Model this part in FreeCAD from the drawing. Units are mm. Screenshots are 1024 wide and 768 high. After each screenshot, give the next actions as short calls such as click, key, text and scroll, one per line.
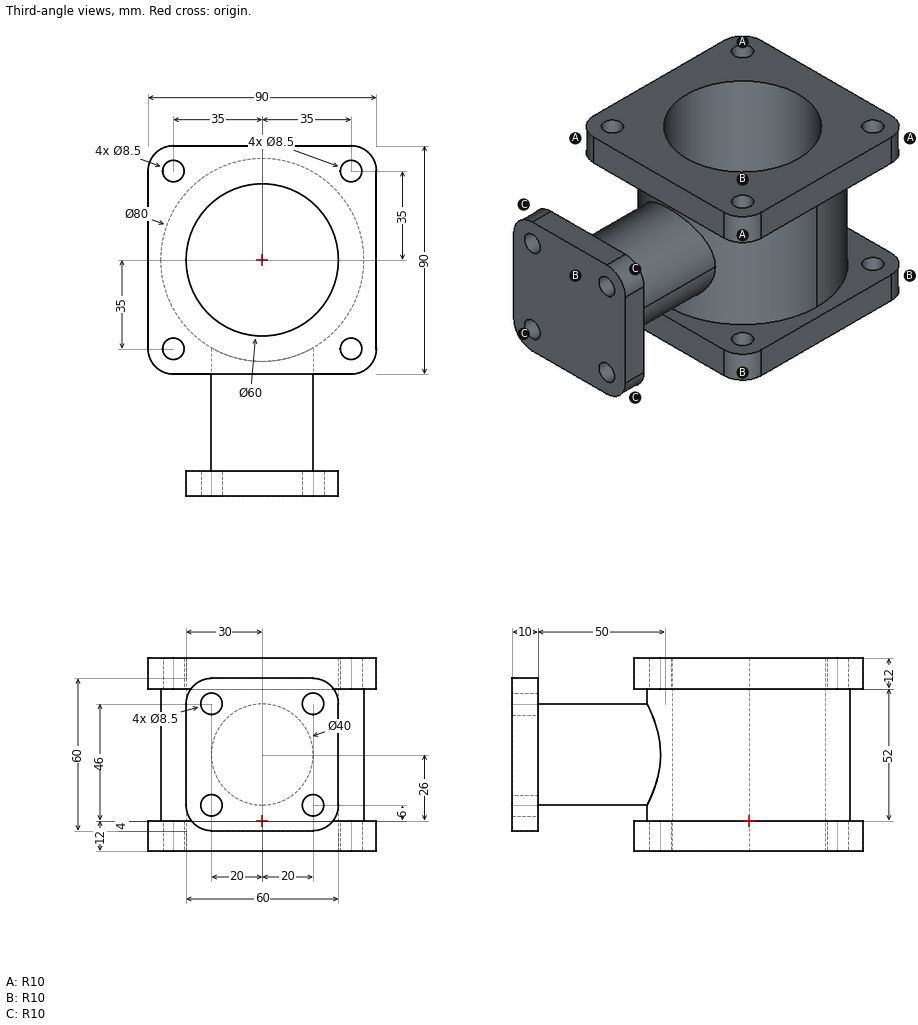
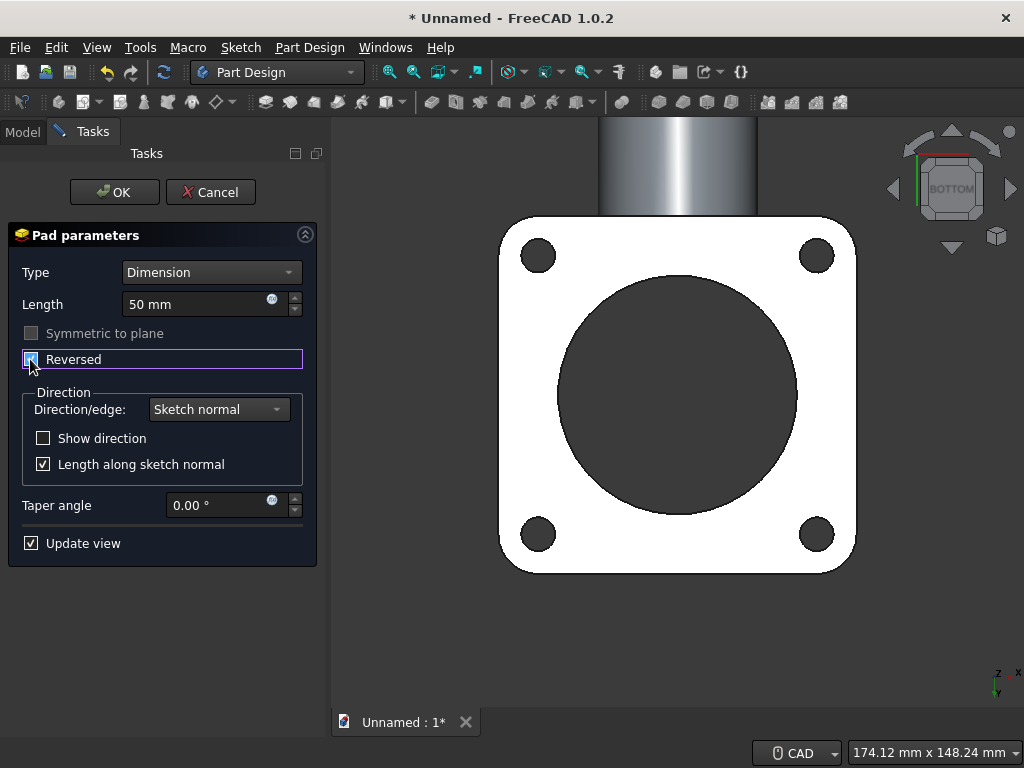
click(115, 192)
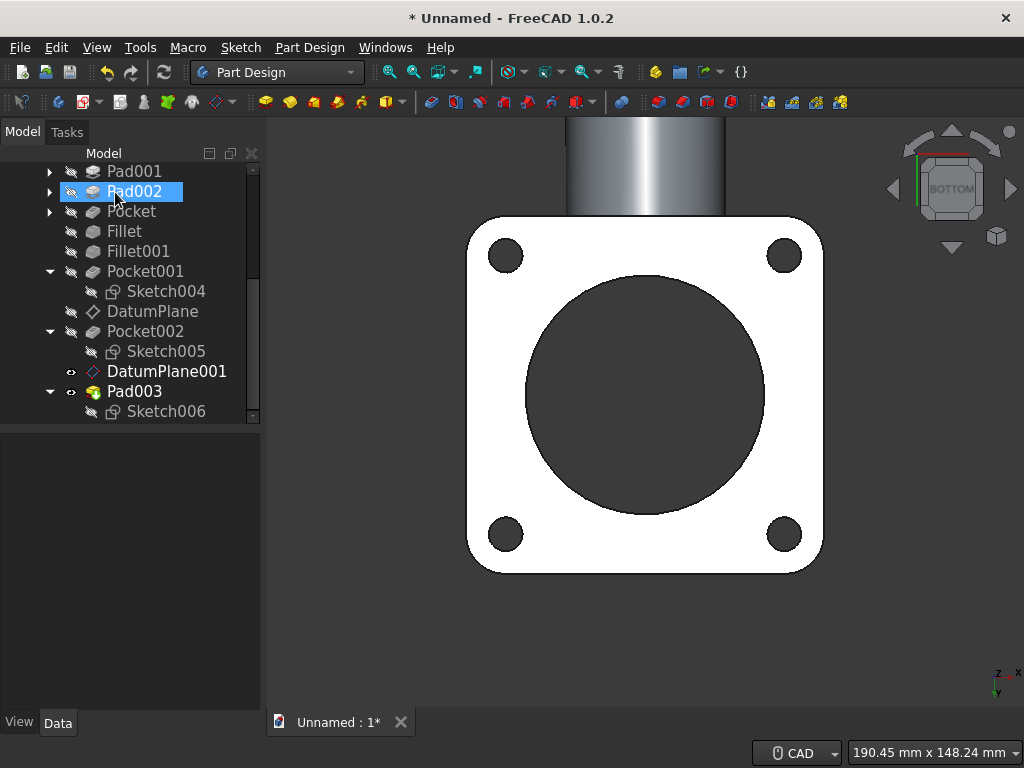
click(116, 372)
key(space)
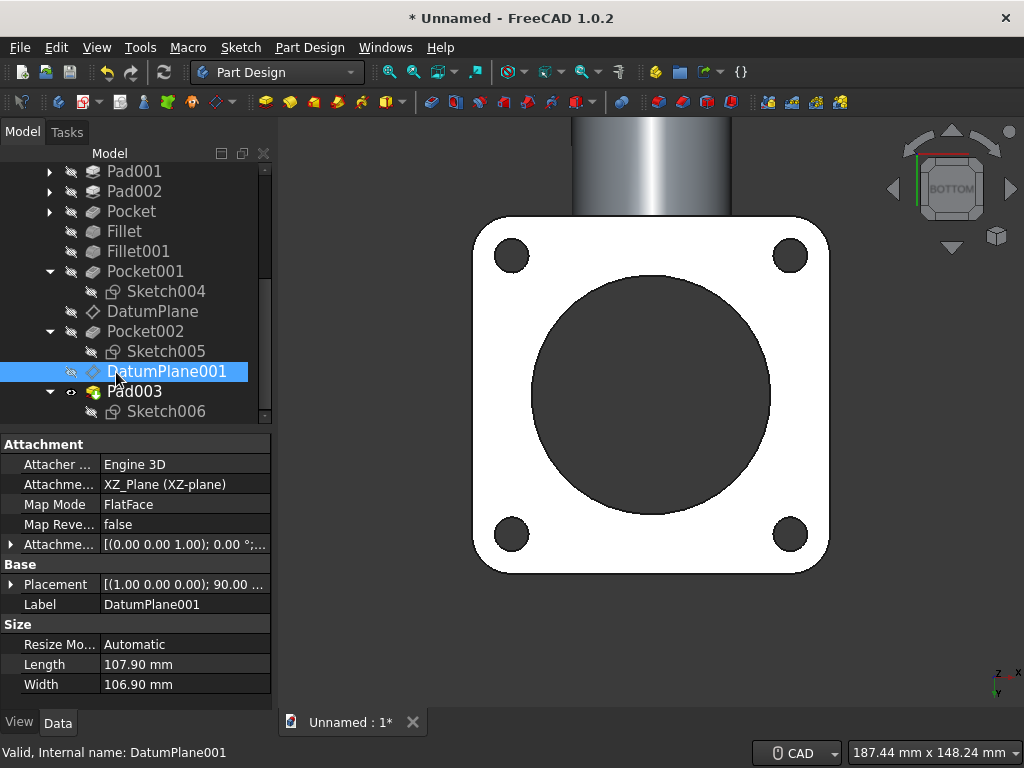
click(390, 72)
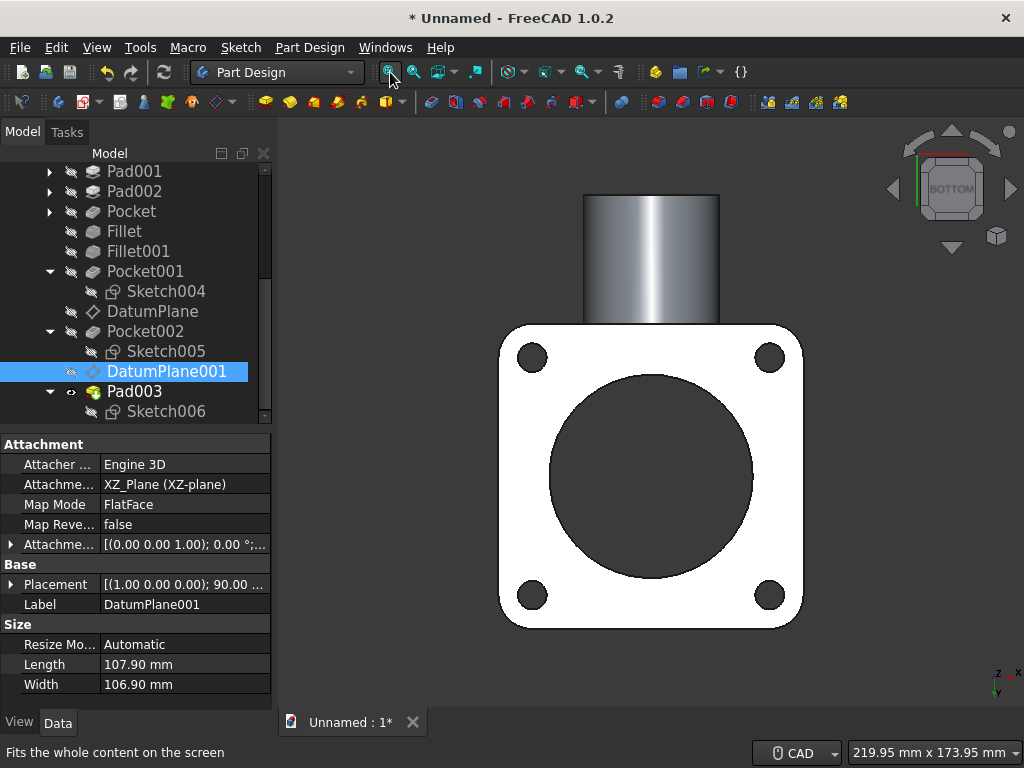
key(0)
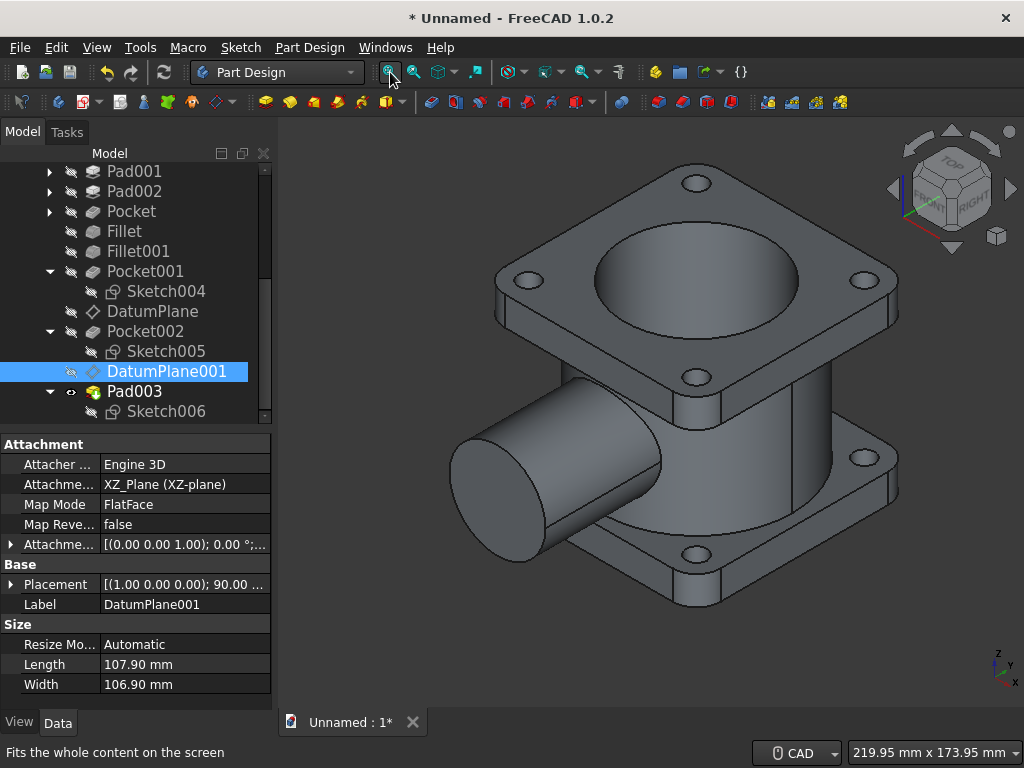
click(498, 500)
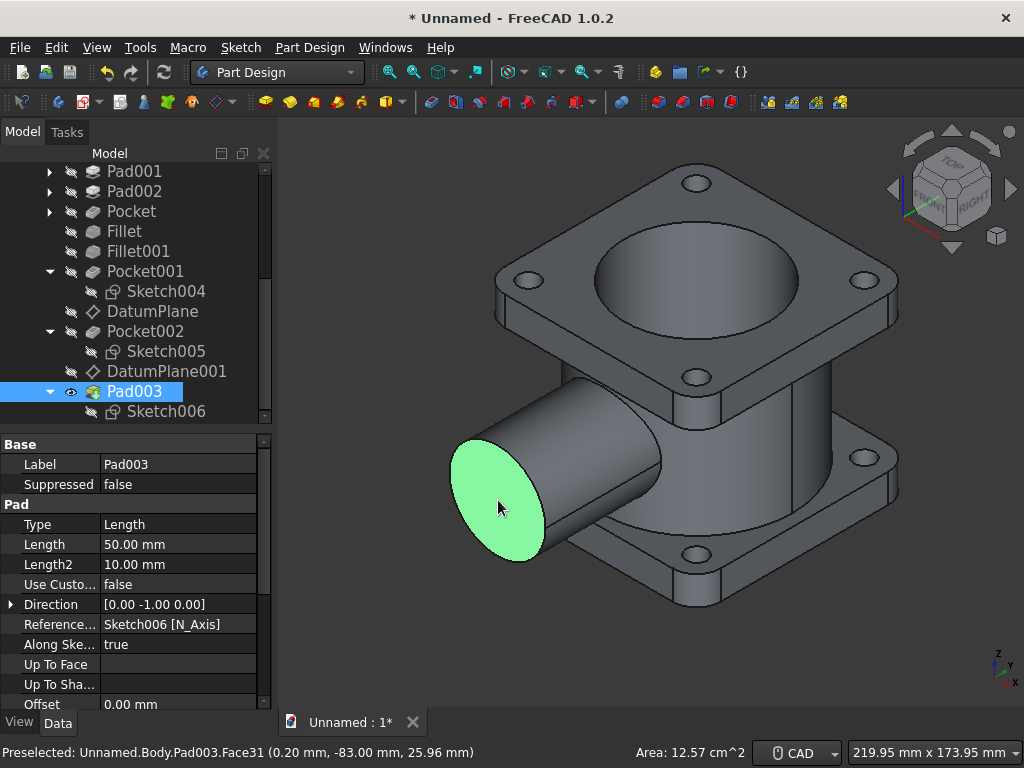
click(84, 102)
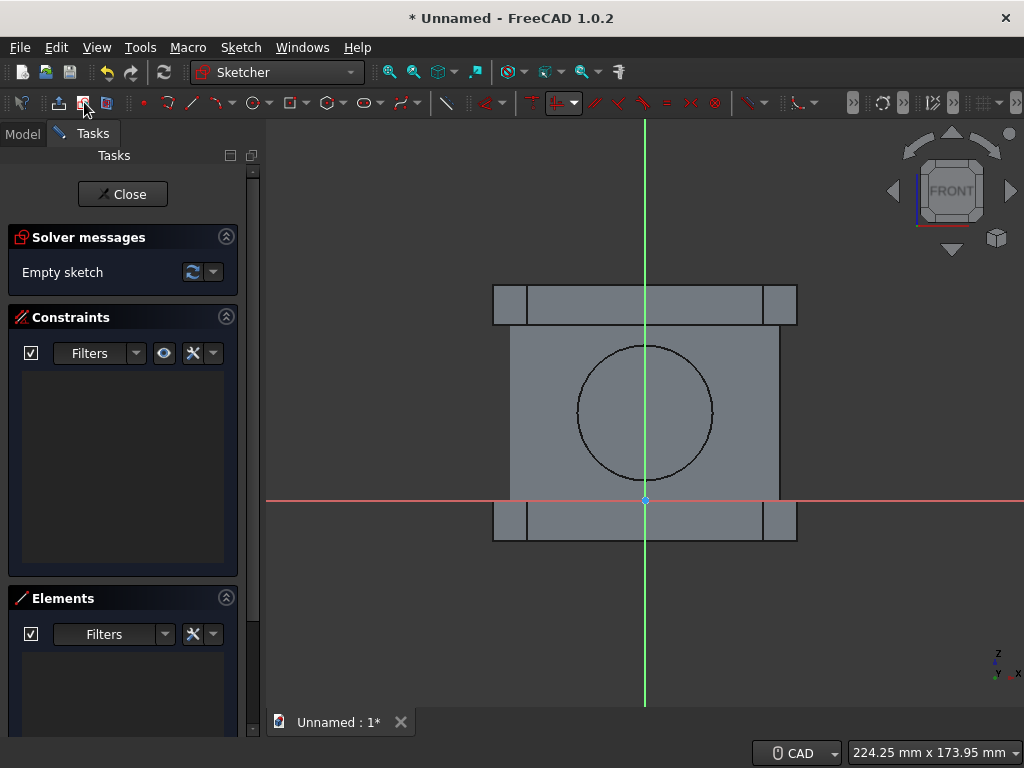
scroll(728, 413, up, 3)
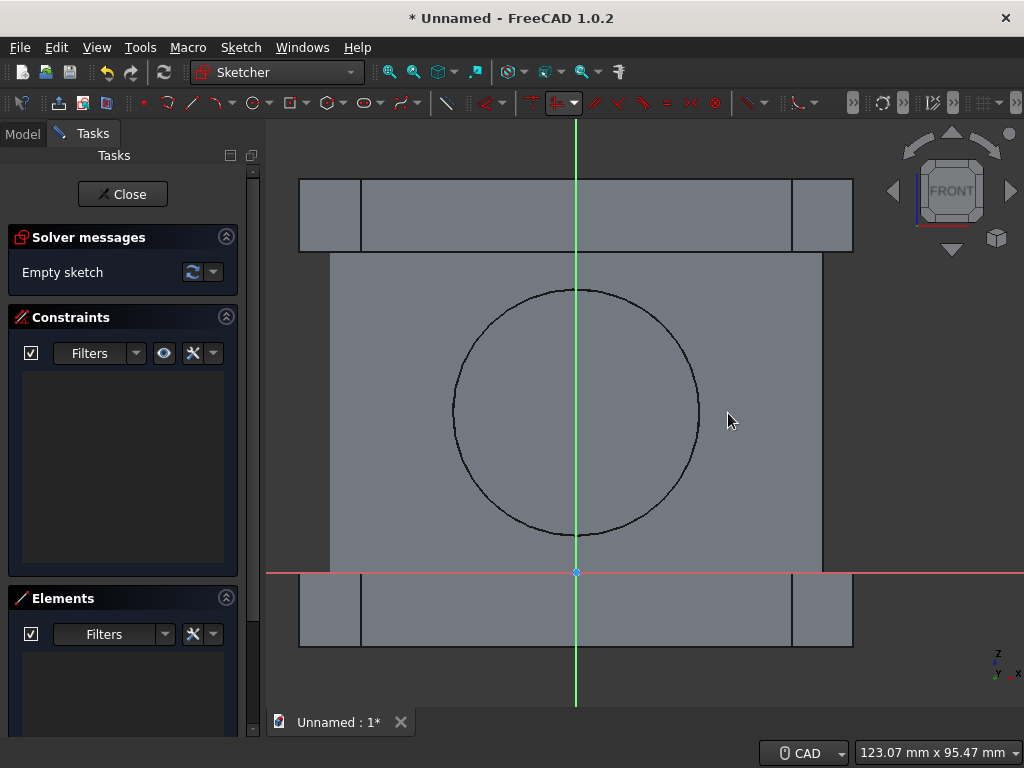
click(308, 104)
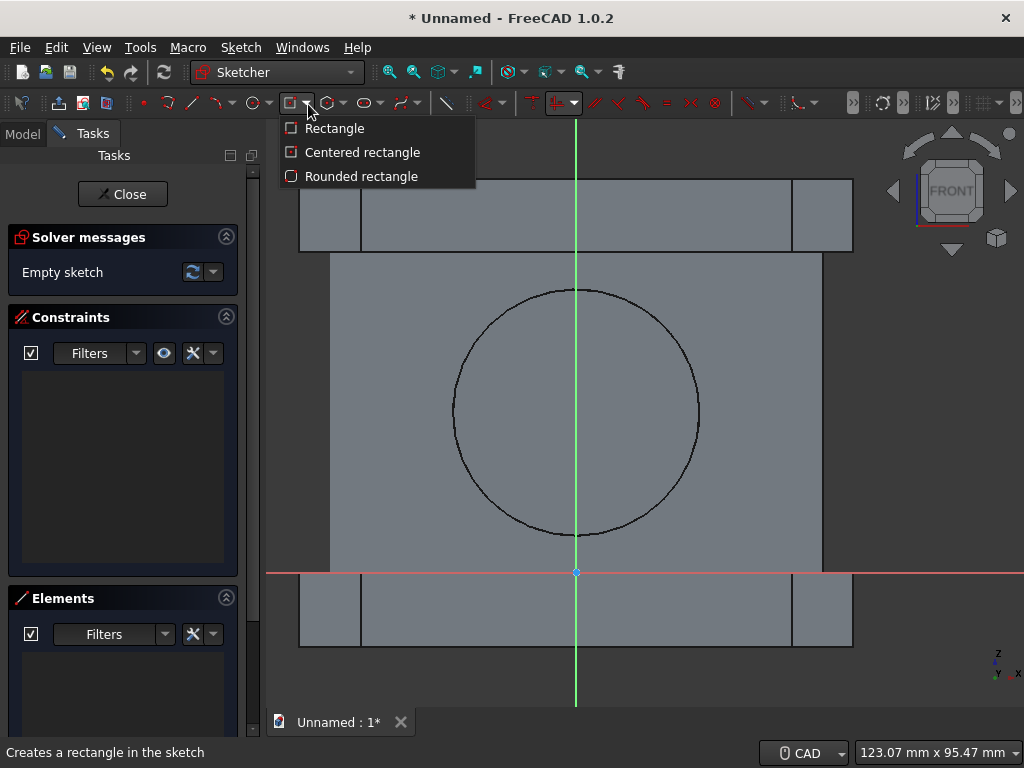
click(378, 128)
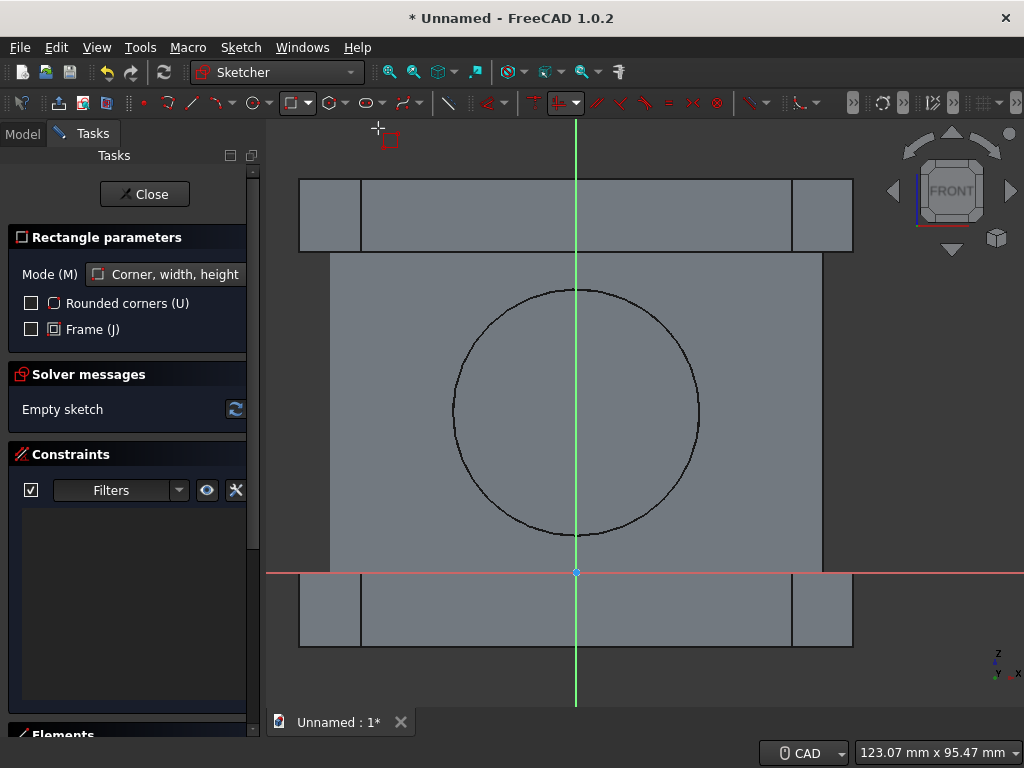
click(391, 228)
click(761, 597)
key(Escape)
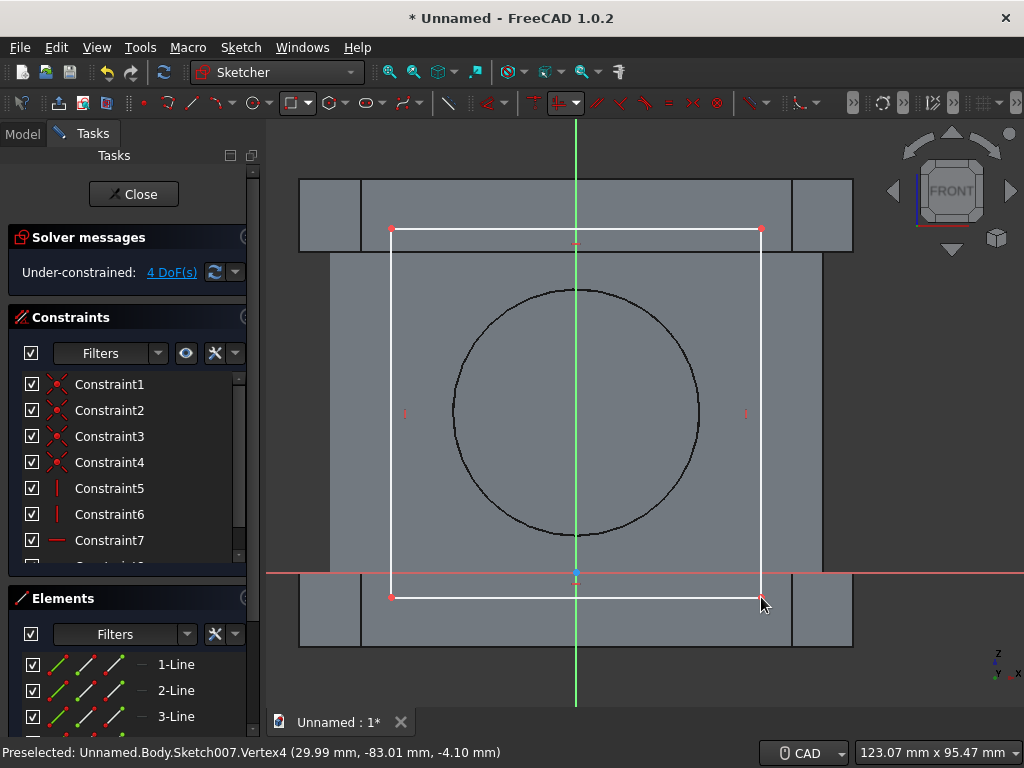
click(488, 104)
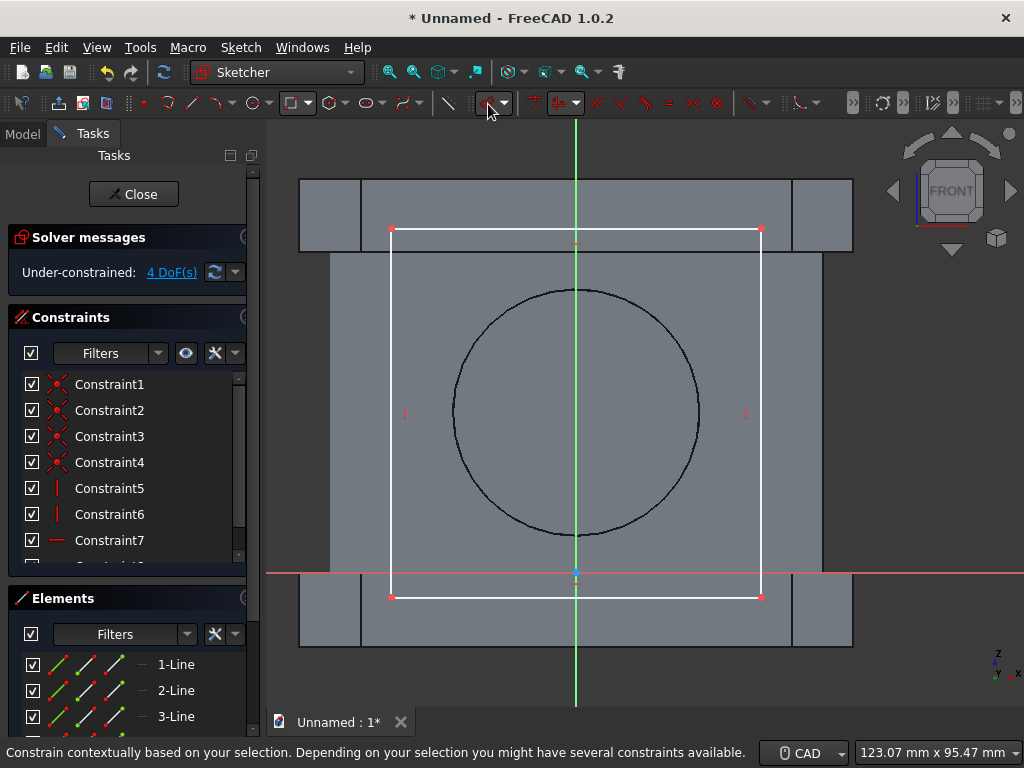
click(391, 340)
click(357, 413)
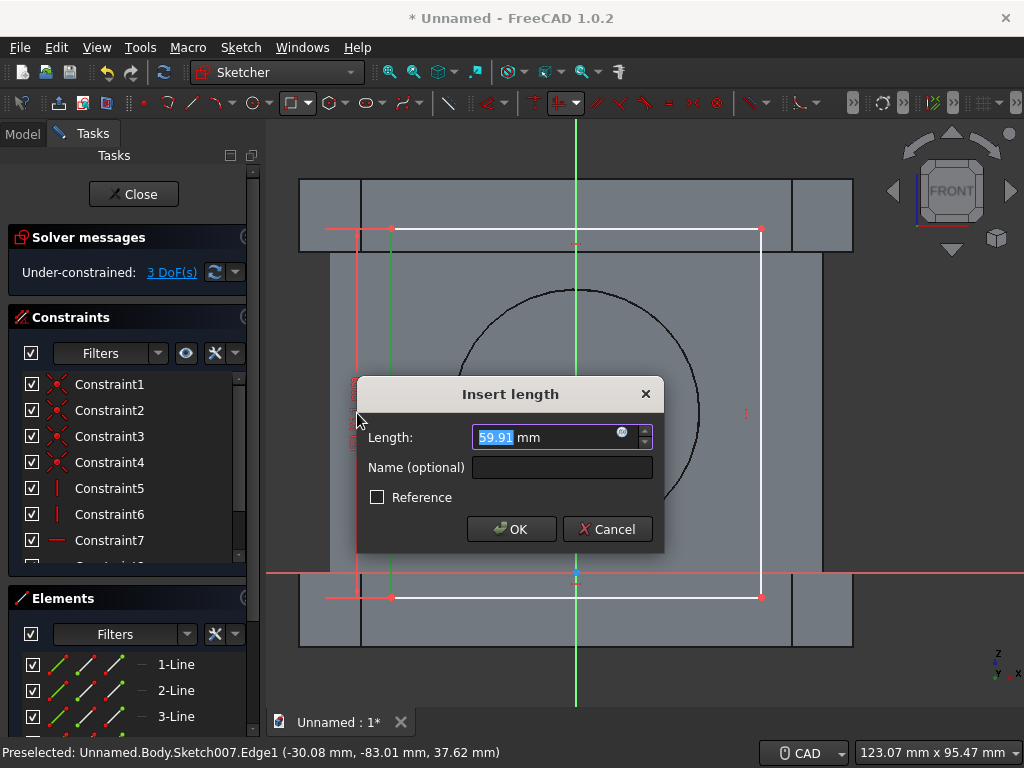
text(60)
key(Return)